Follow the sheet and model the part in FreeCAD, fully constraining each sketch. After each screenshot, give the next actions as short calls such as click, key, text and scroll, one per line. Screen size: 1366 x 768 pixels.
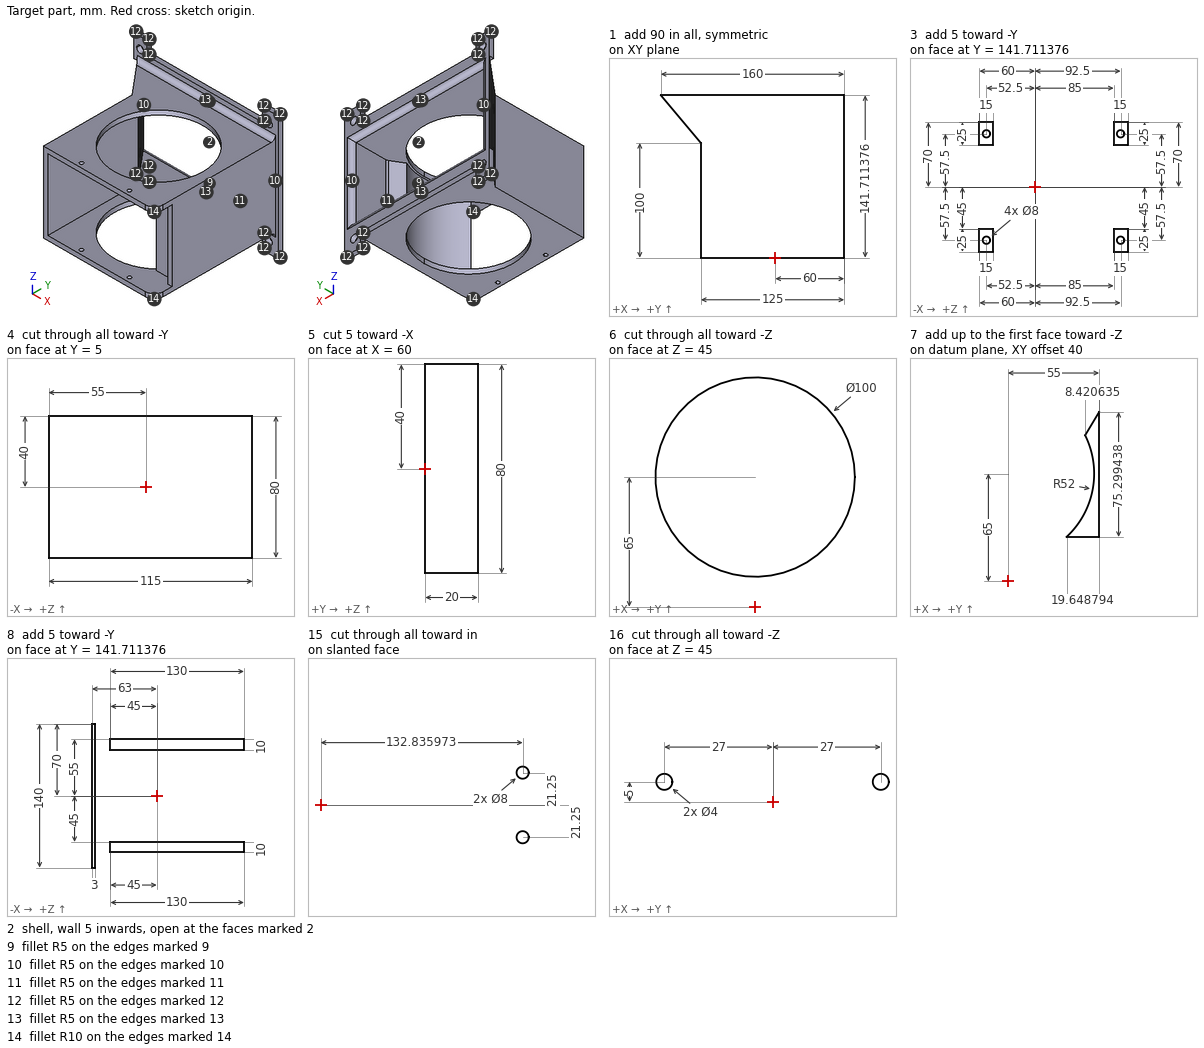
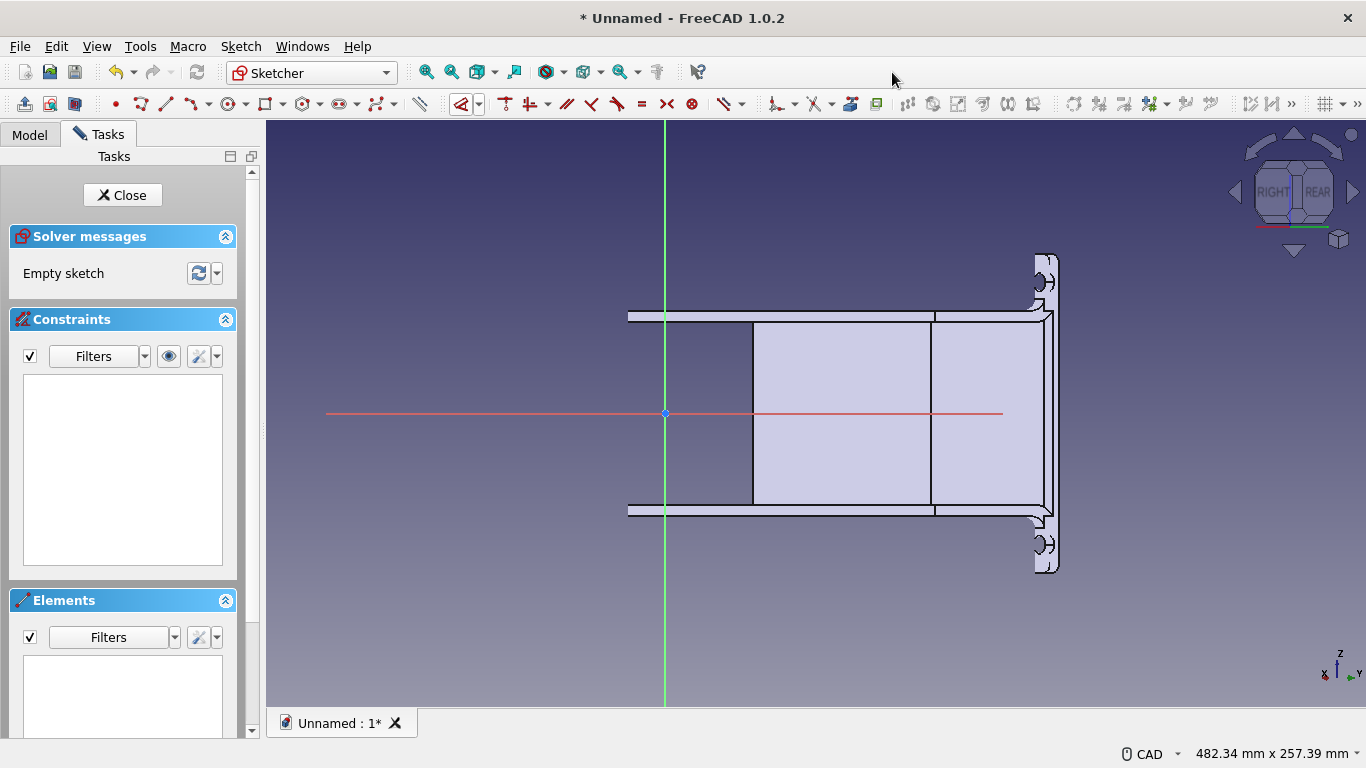
scroll(1063, 413, up, 6)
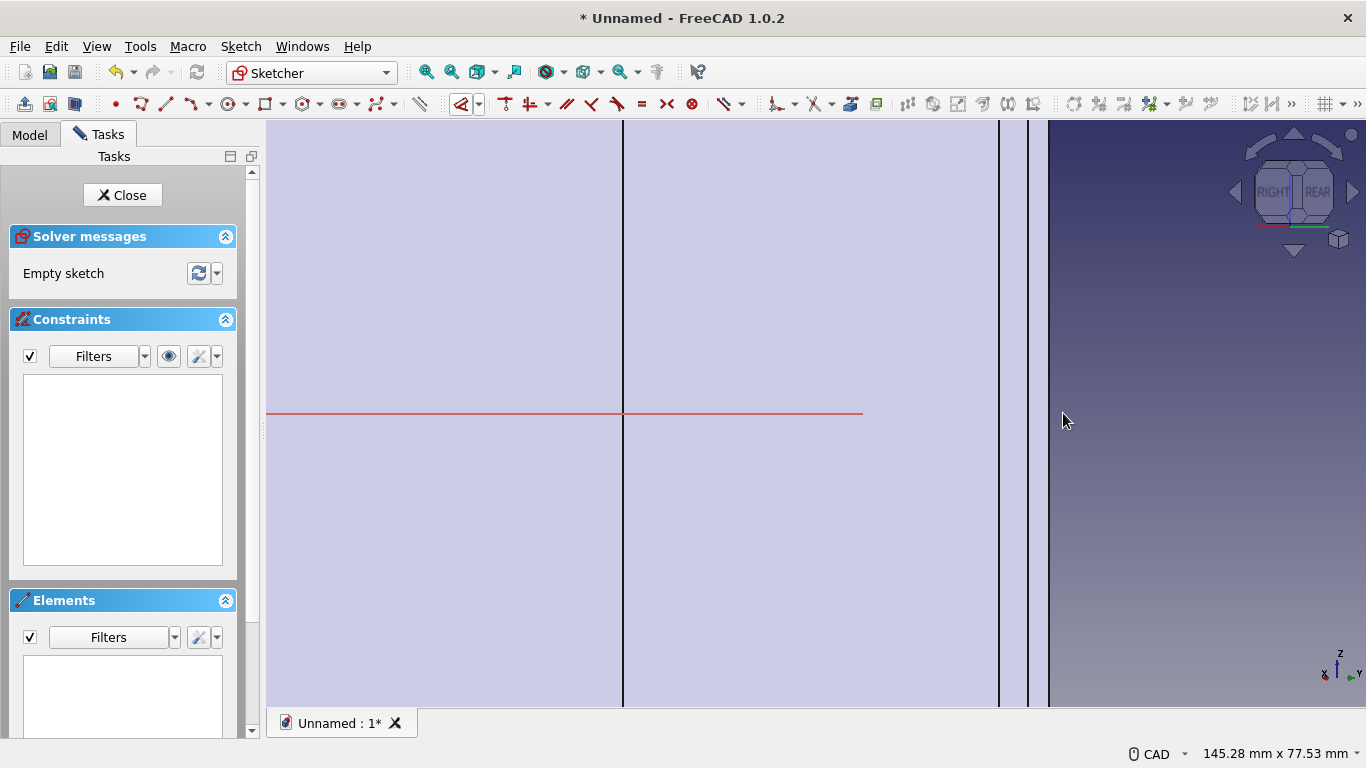
key(g)
key(c)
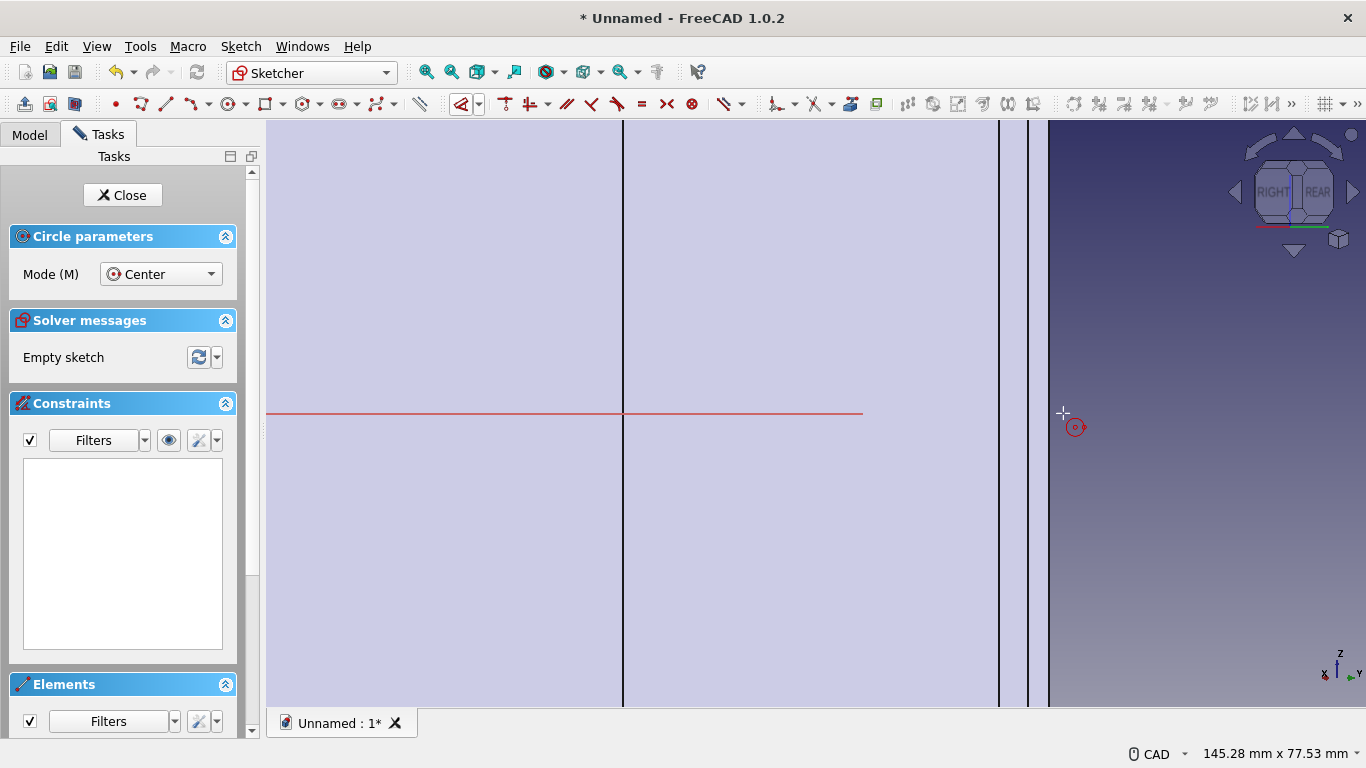
click(746, 253)
move(767, 231)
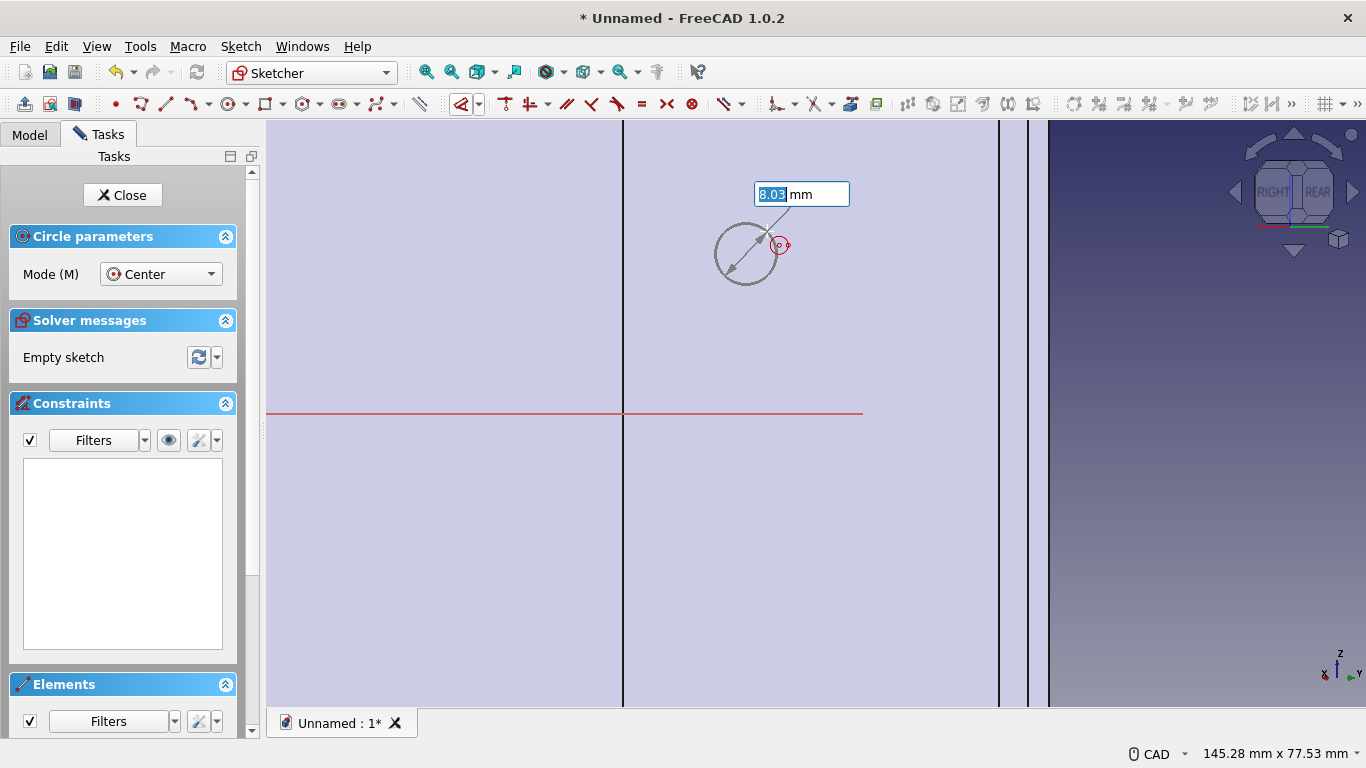
text(8)
key(Return)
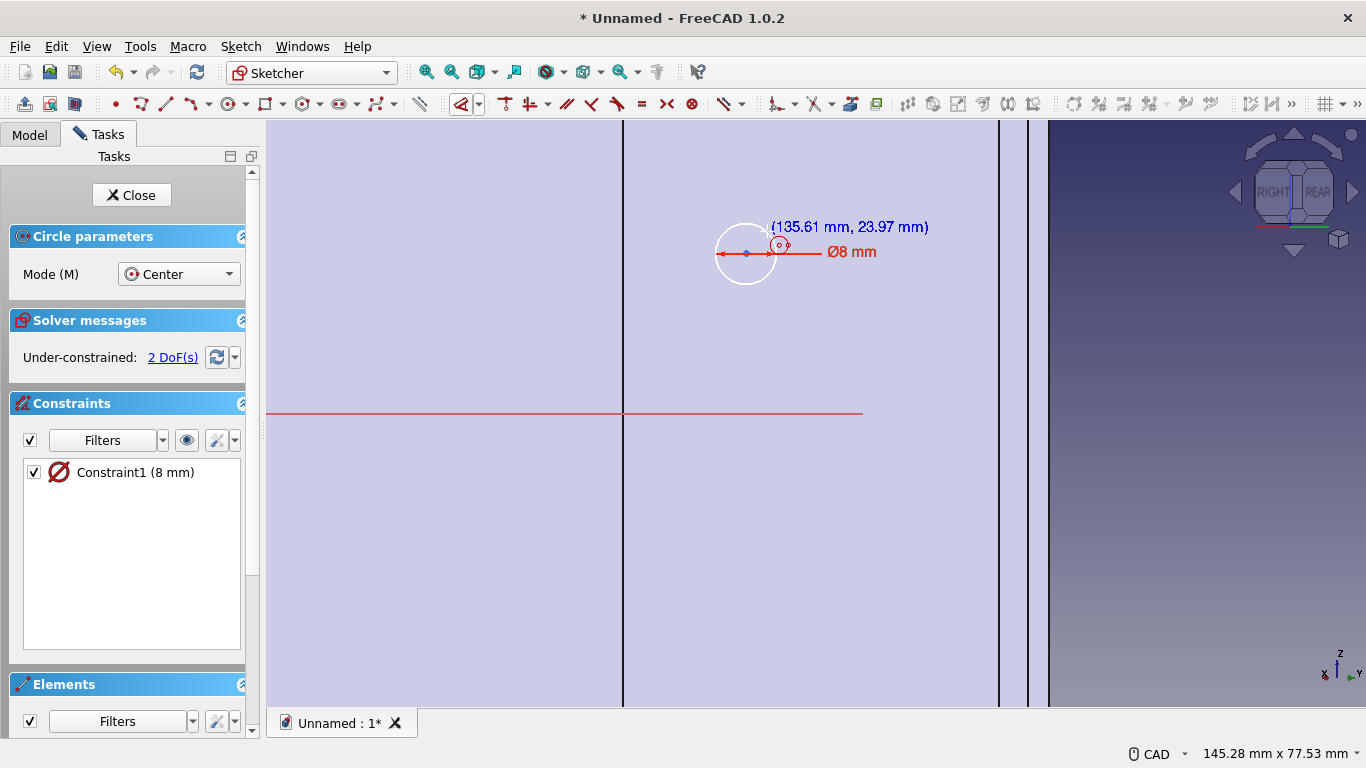
click(746, 574)
move(767, 553)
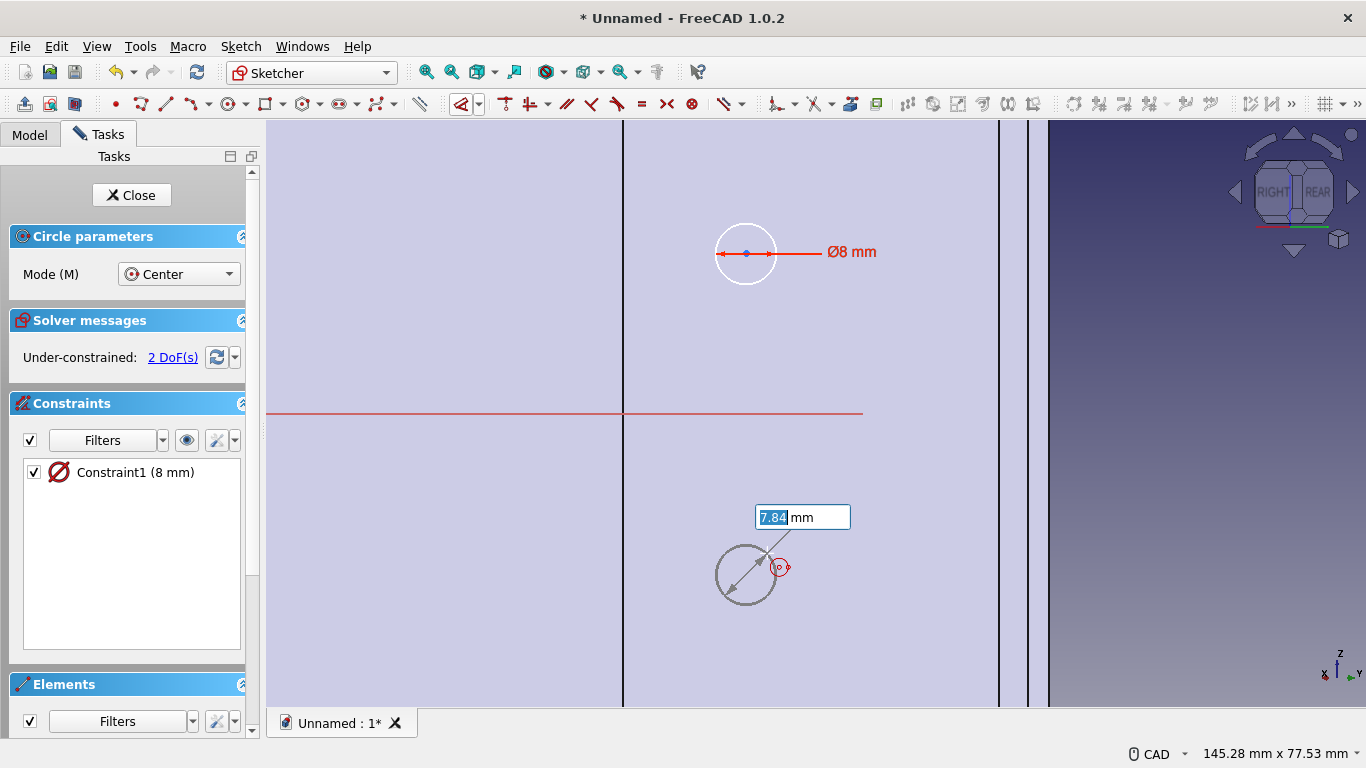
text(8)
key(Return)
key(Escape)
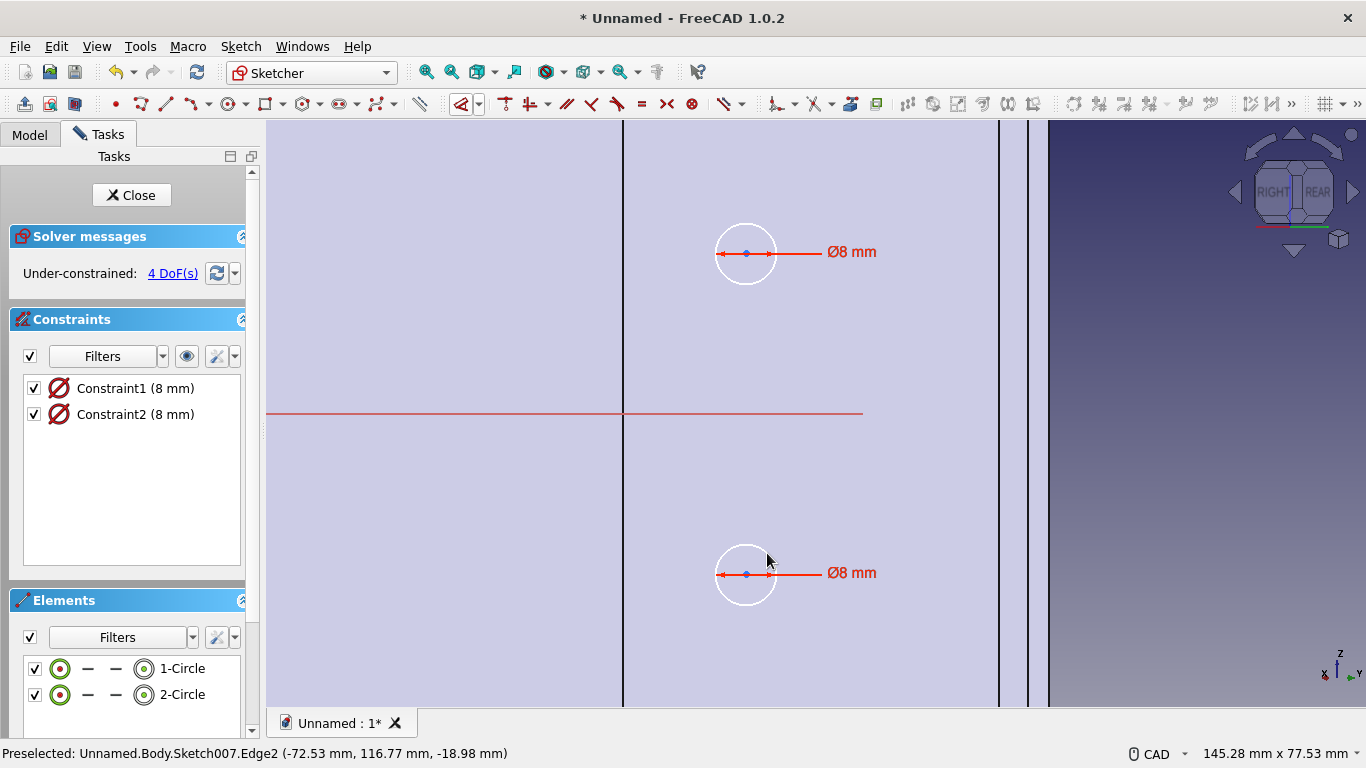
click(746, 254)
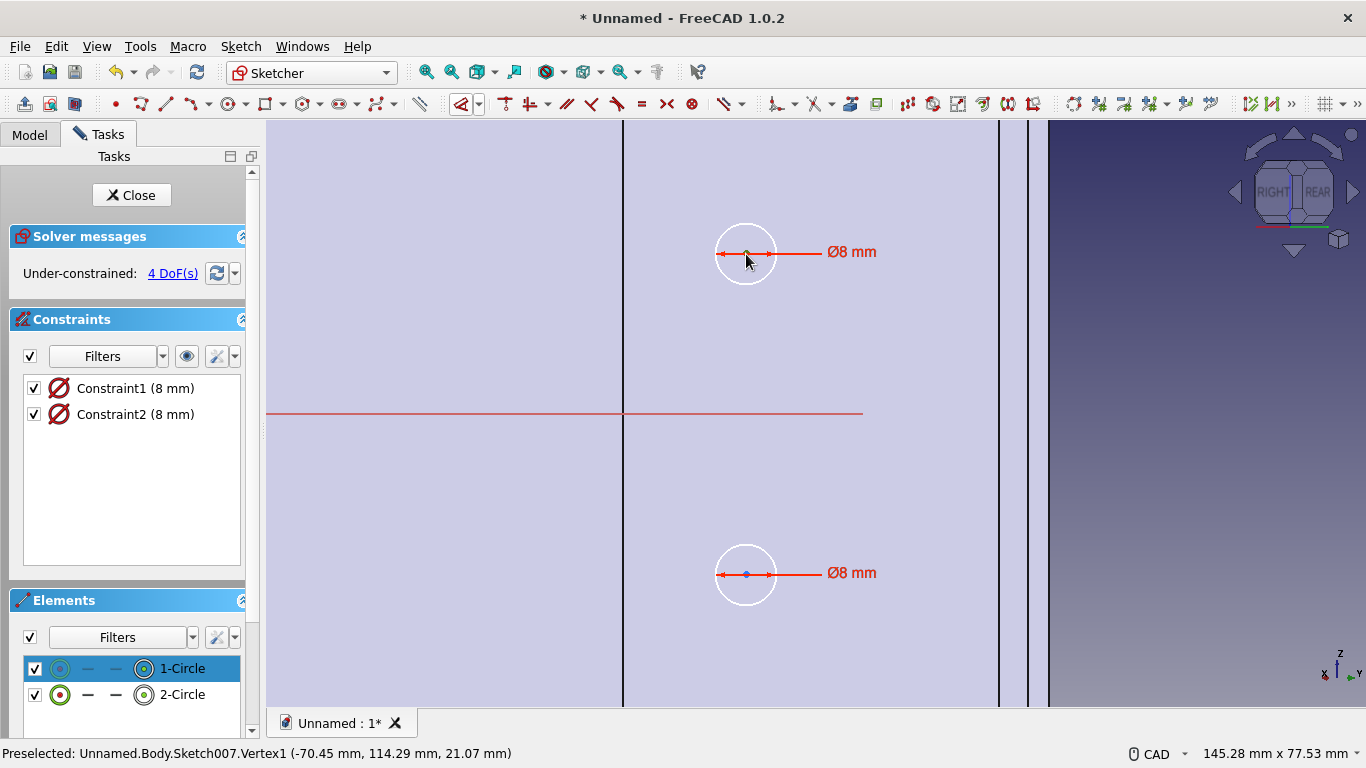
click(746, 575)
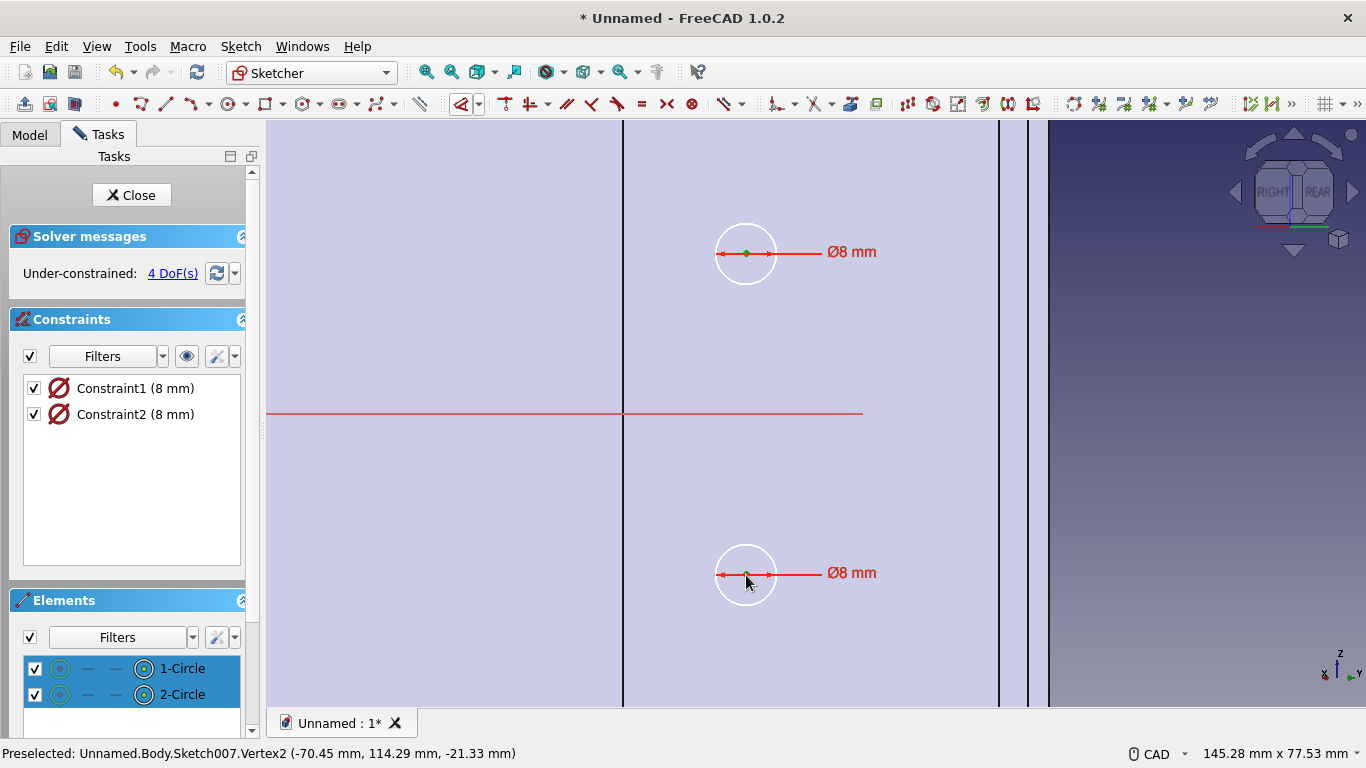
key(v)